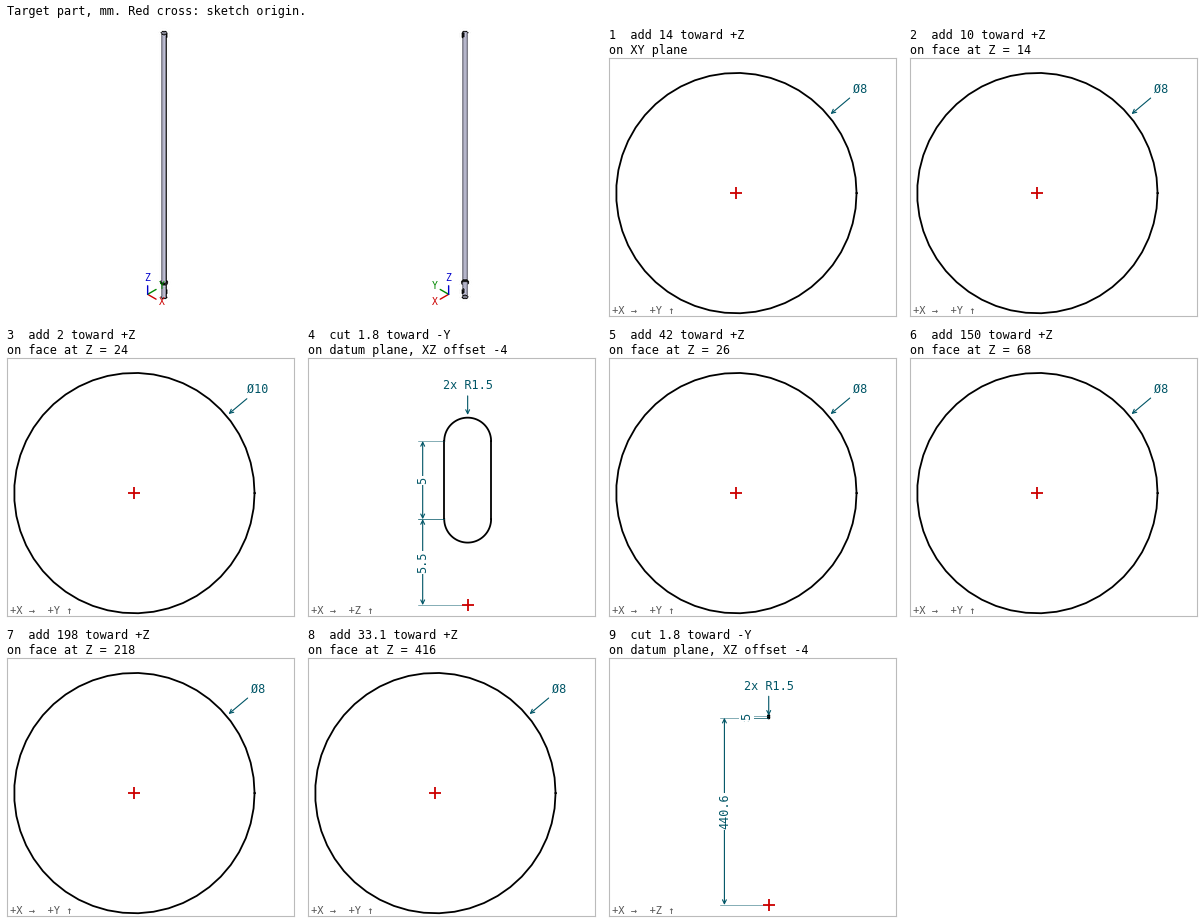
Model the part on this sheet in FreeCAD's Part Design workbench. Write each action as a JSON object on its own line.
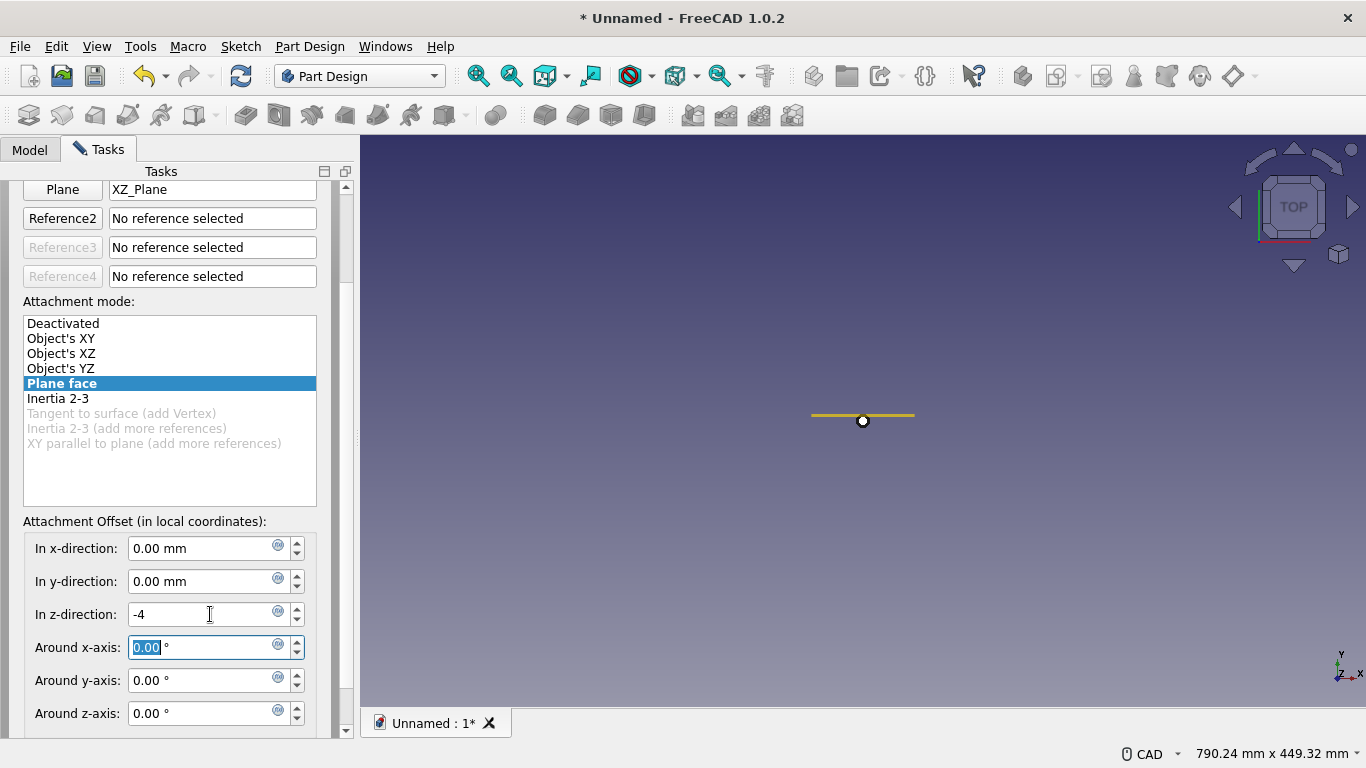
{"action": "scroll", "coordinate": [346, 460], "scroll_direction": "up", "scroll_amount": 3}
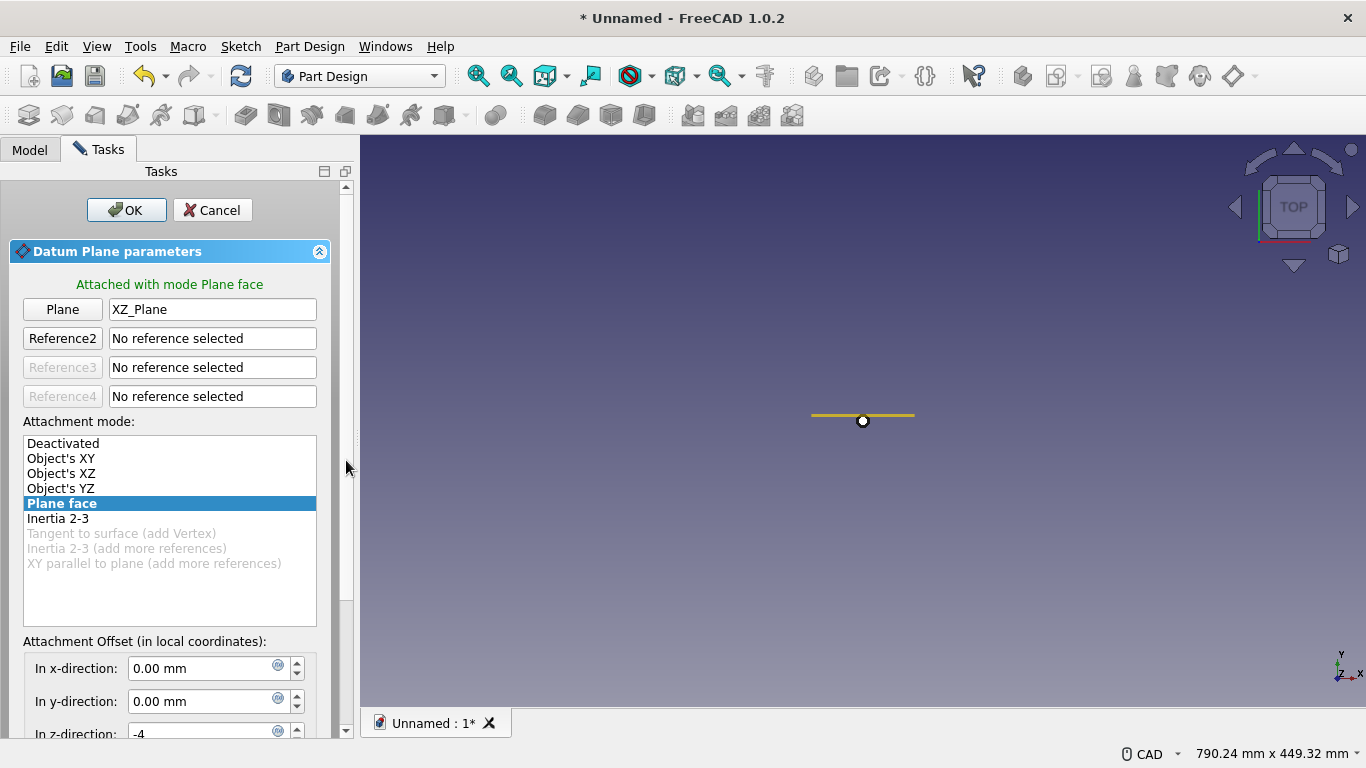
{"action": "left_click", "coordinate": [127, 210]}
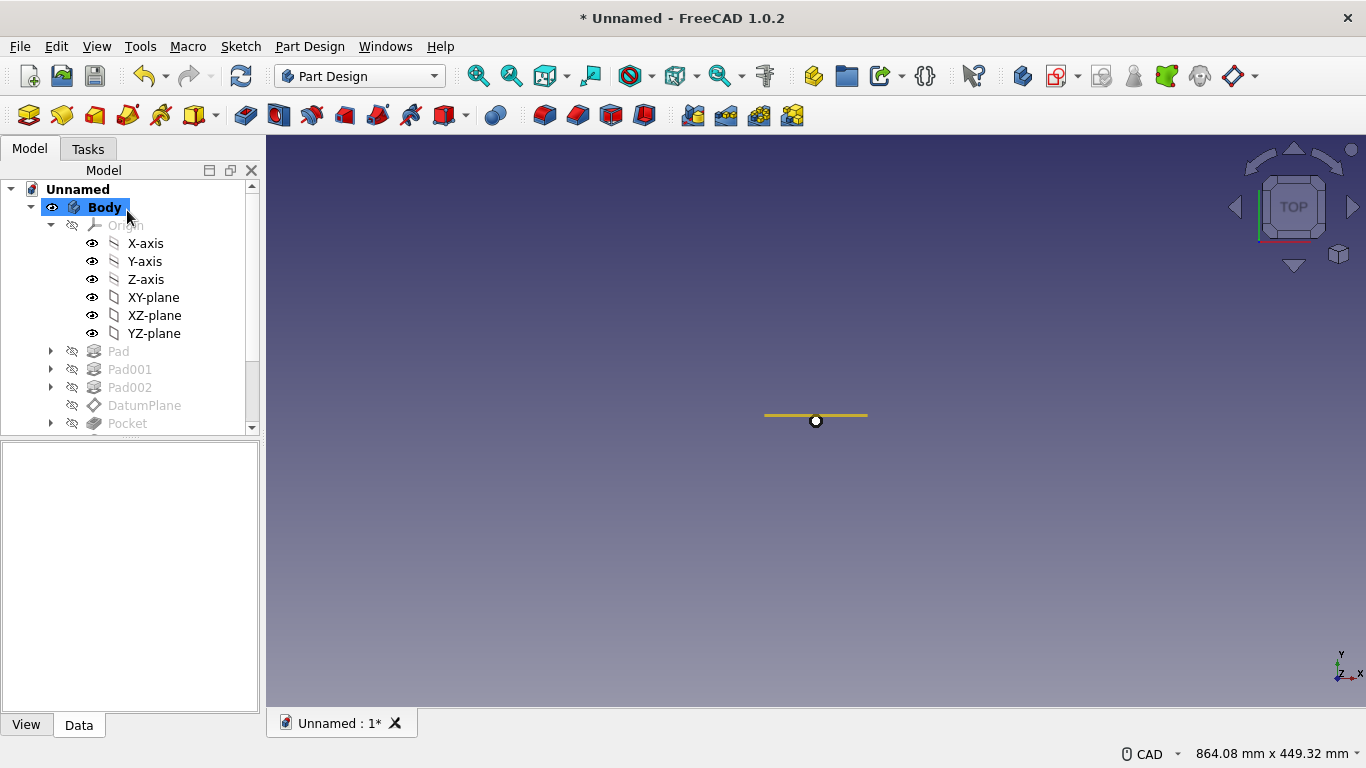
{"action": "scroll", "coordinate": [101, 311], "scroll_direction": "down", "scroll_amount": 3}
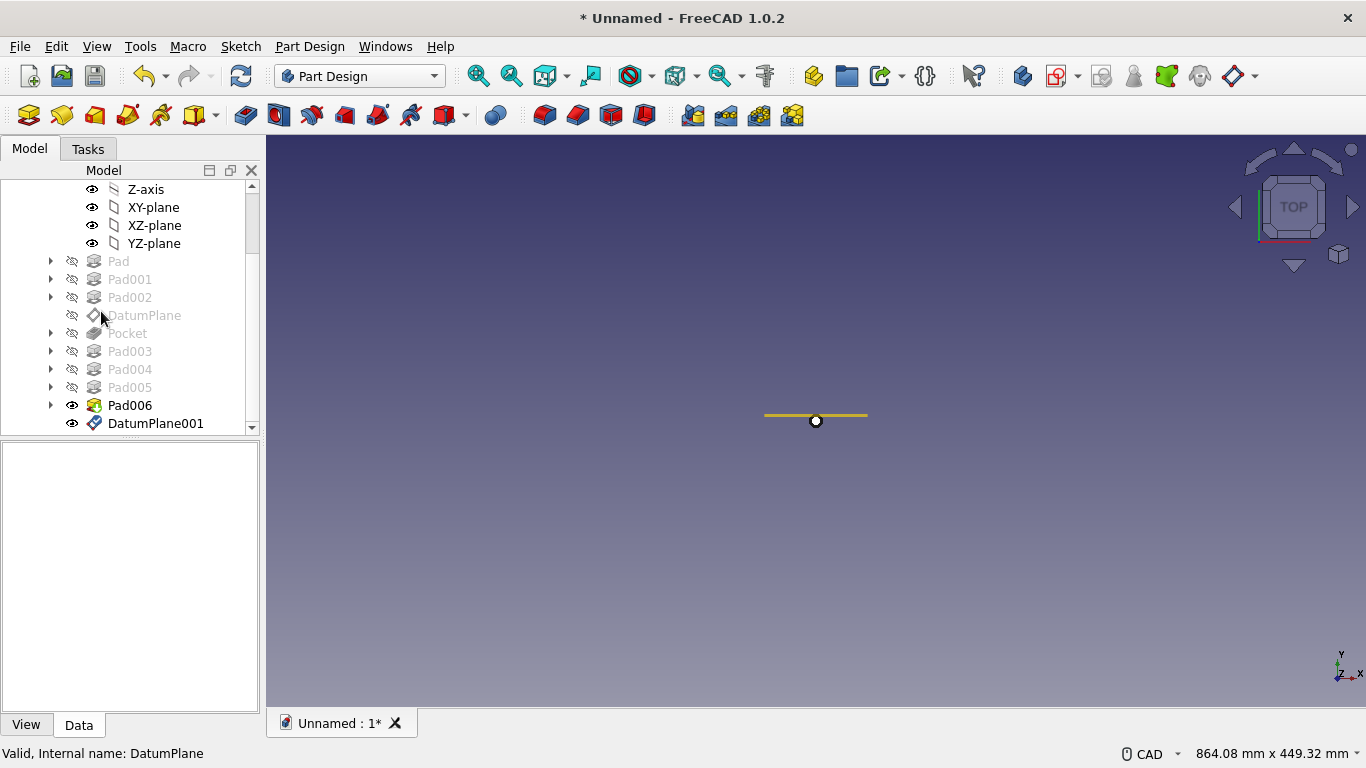
{"action": "left_click", "coordinate": [117, 423]}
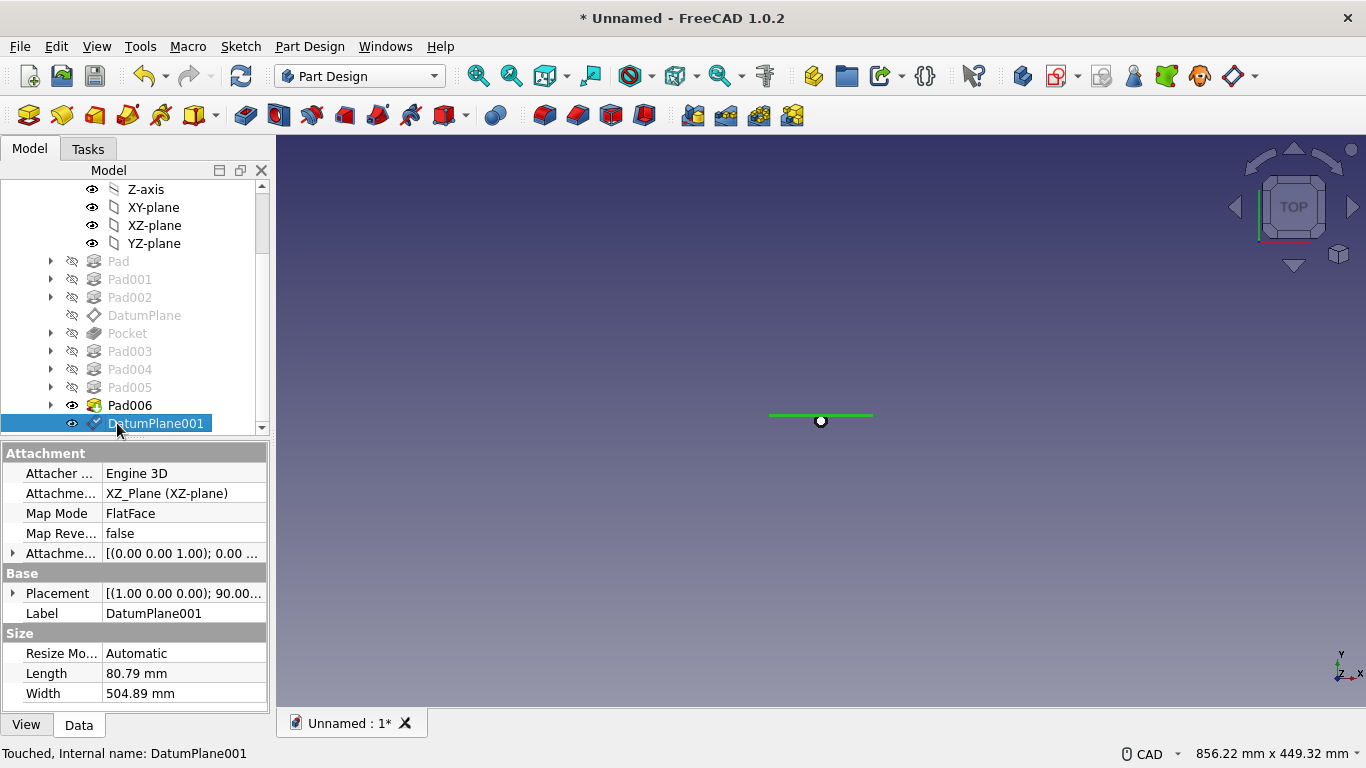
{"action": "left_click", "coordinate": [1056, 76]}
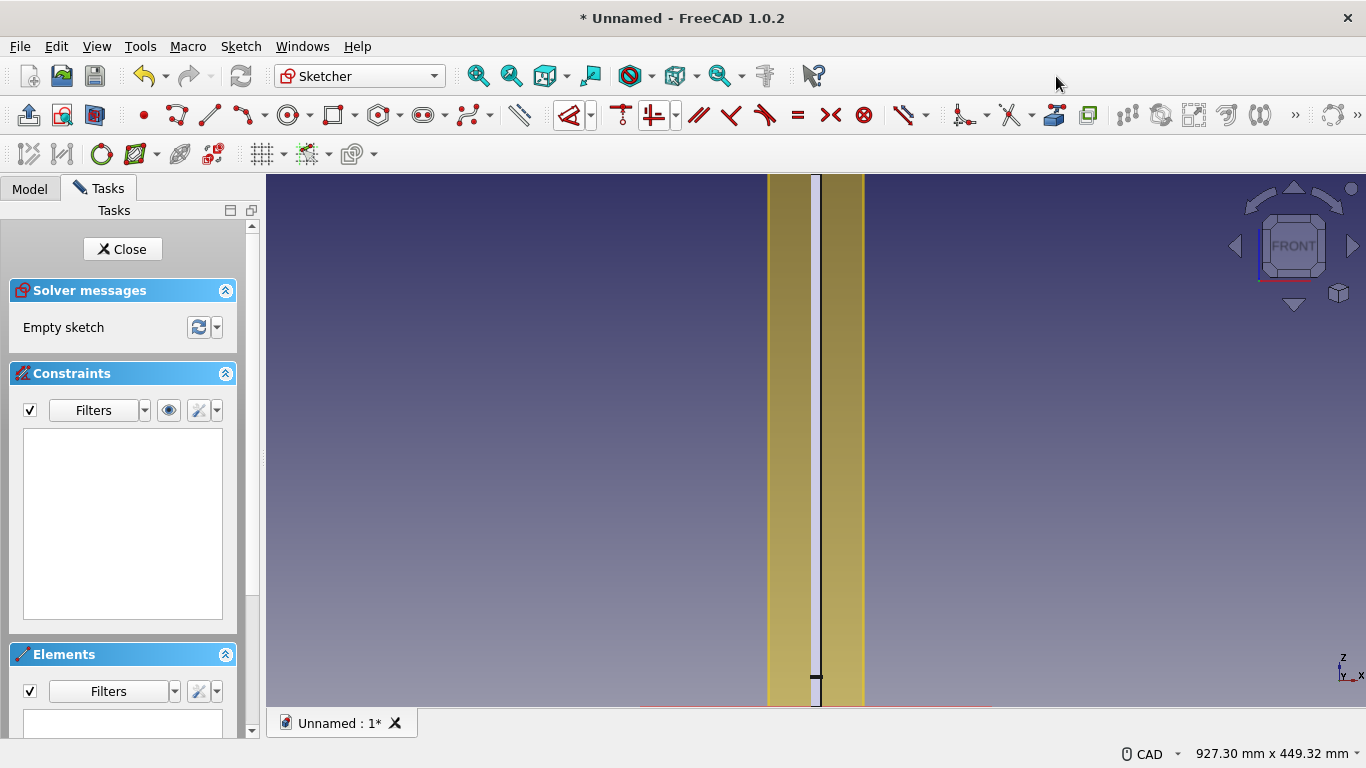
{"action": "left_click", "coordinate": [95, 116]}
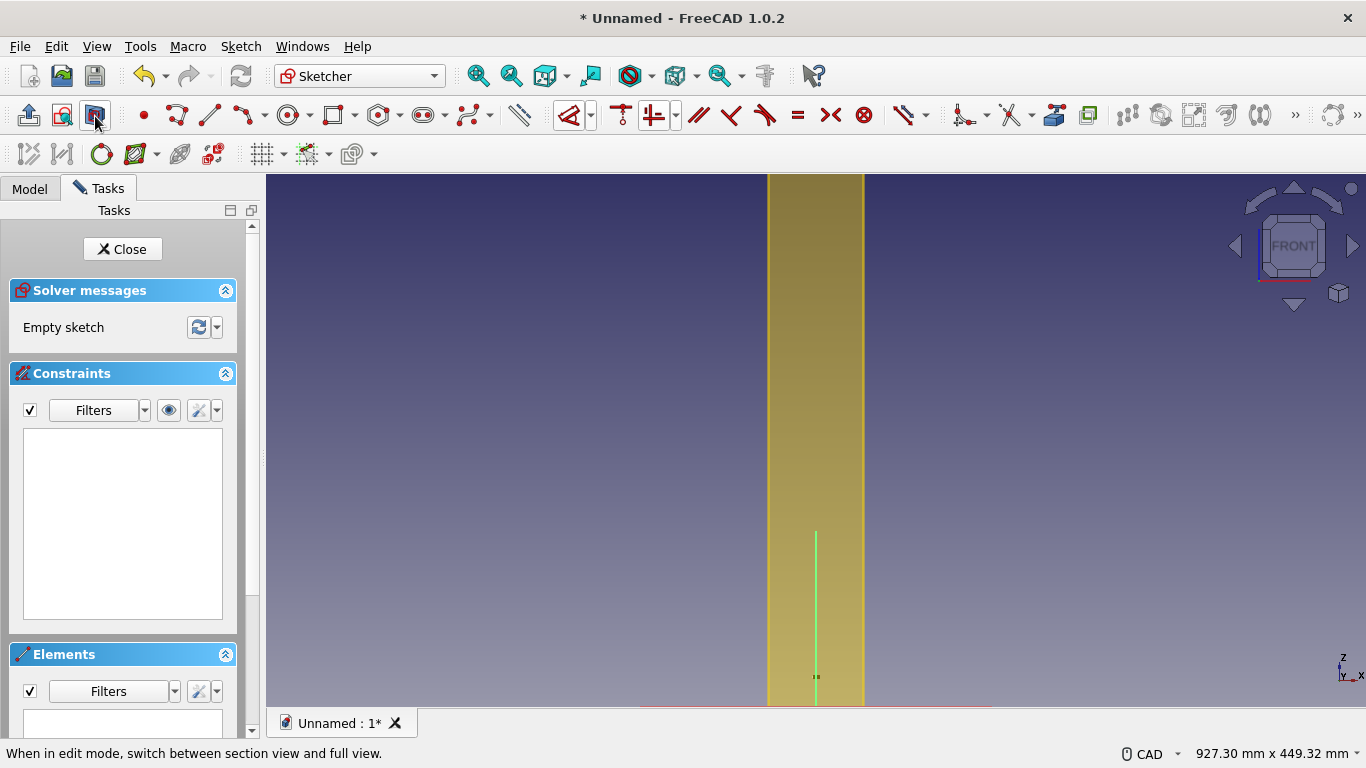
{"action": "scroll", "coordinate": [748, 440], "scroll_direction": "down", "scroll_amount": 5}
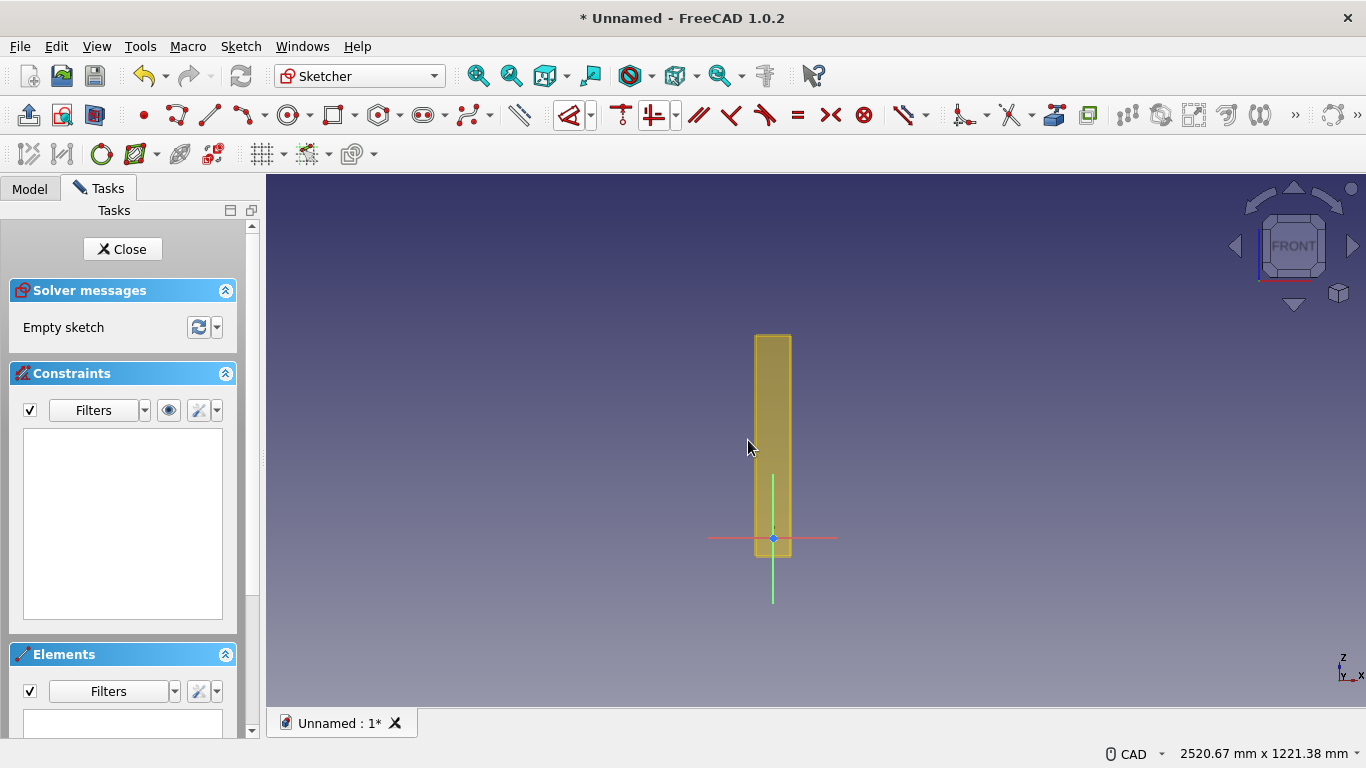
{"action": "scroll", "coordinate": [775, 340], "scroll_direction": "up", "scroll_amount": 15}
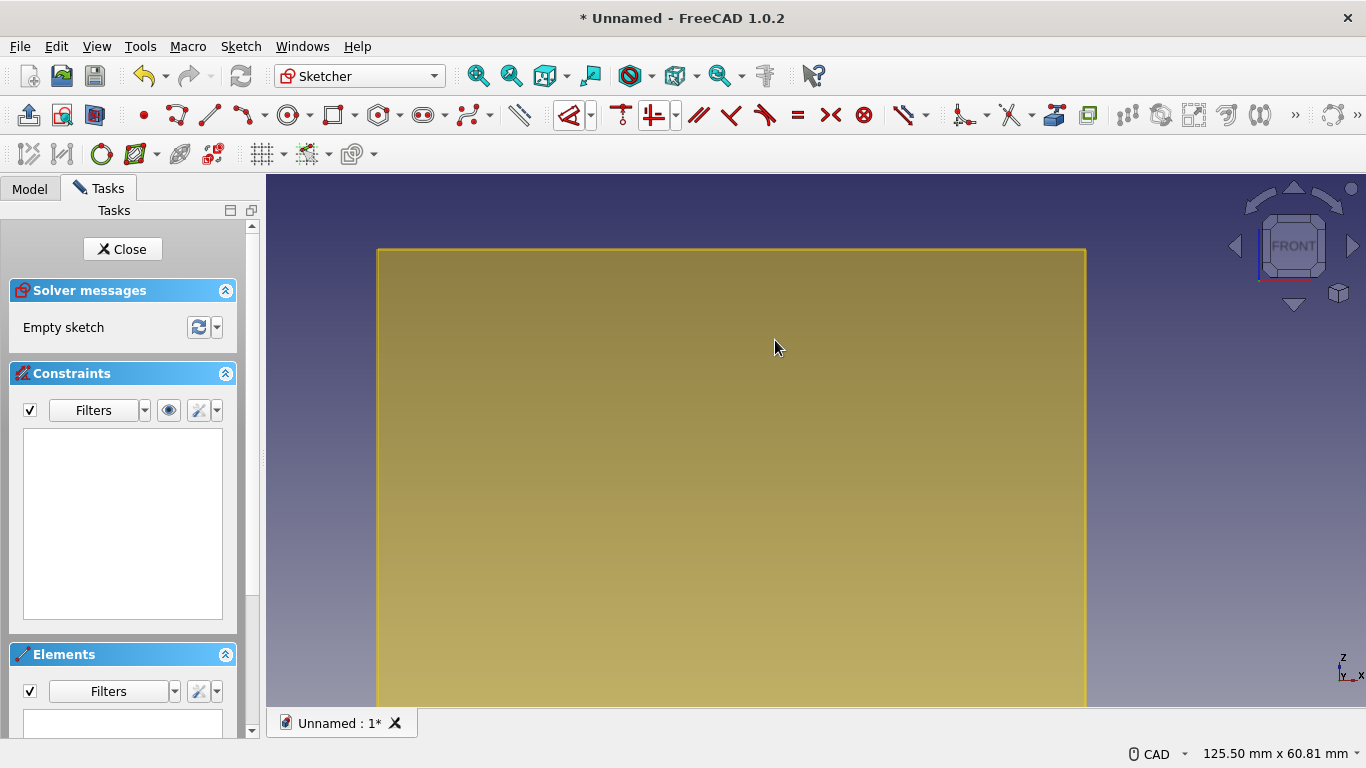
{"action": "scroll", "coordinate": [728, 436], "scroll_direction": "up", "scroll_amount": 8}